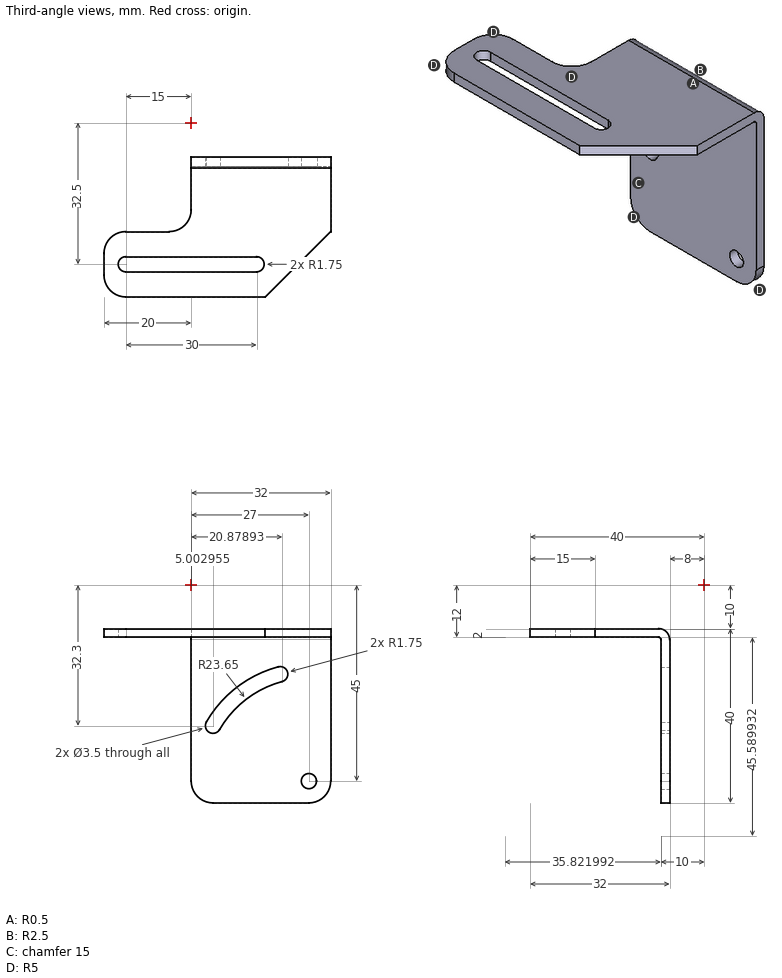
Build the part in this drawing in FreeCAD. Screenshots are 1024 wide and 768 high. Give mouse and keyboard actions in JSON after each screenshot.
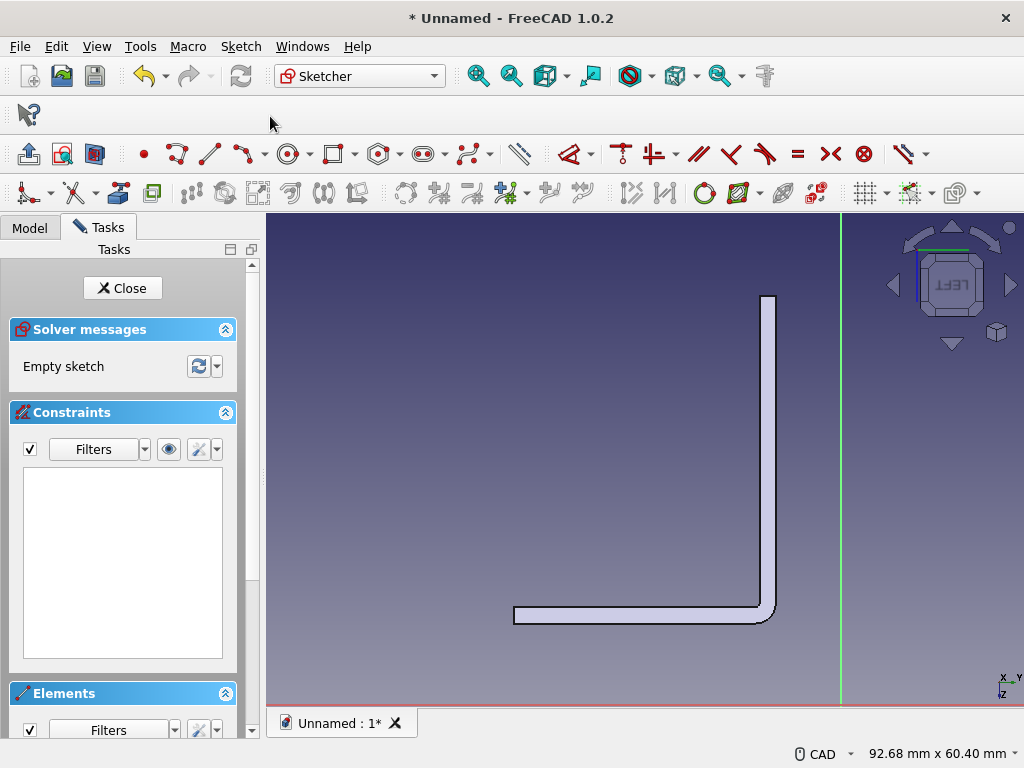
{"action": "scroll", "coordinate": [575, 679], "scroll_direction": "up", "scroll_amount": 6}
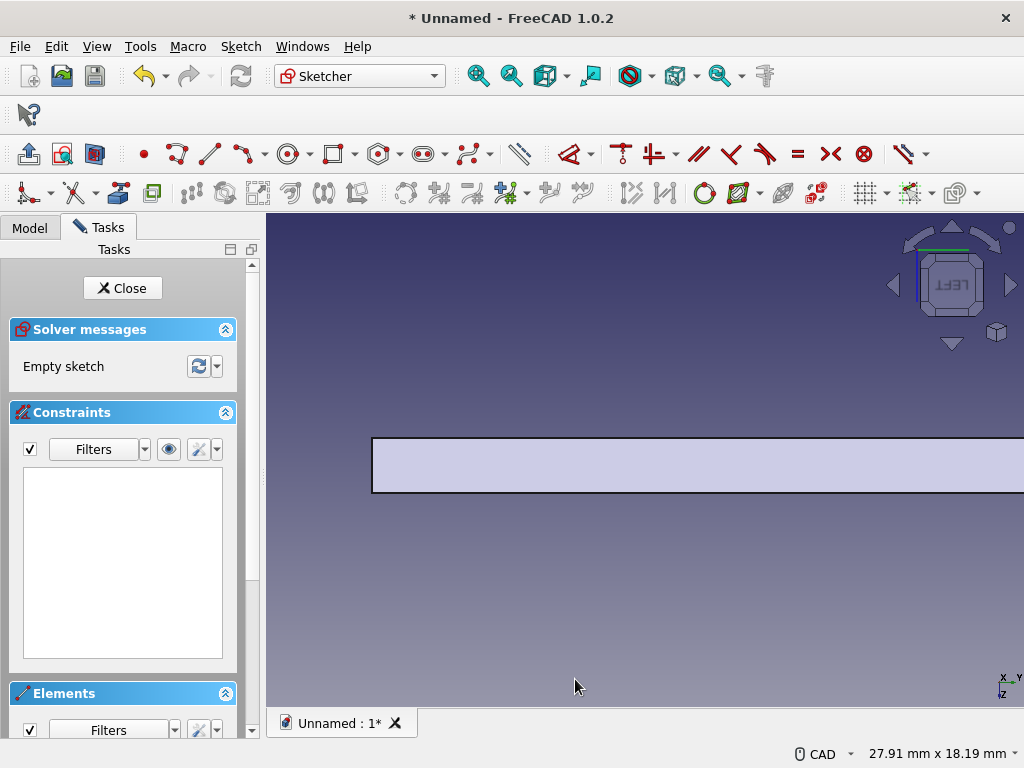
{"action": "left_click", "coordinate": [332, 154]}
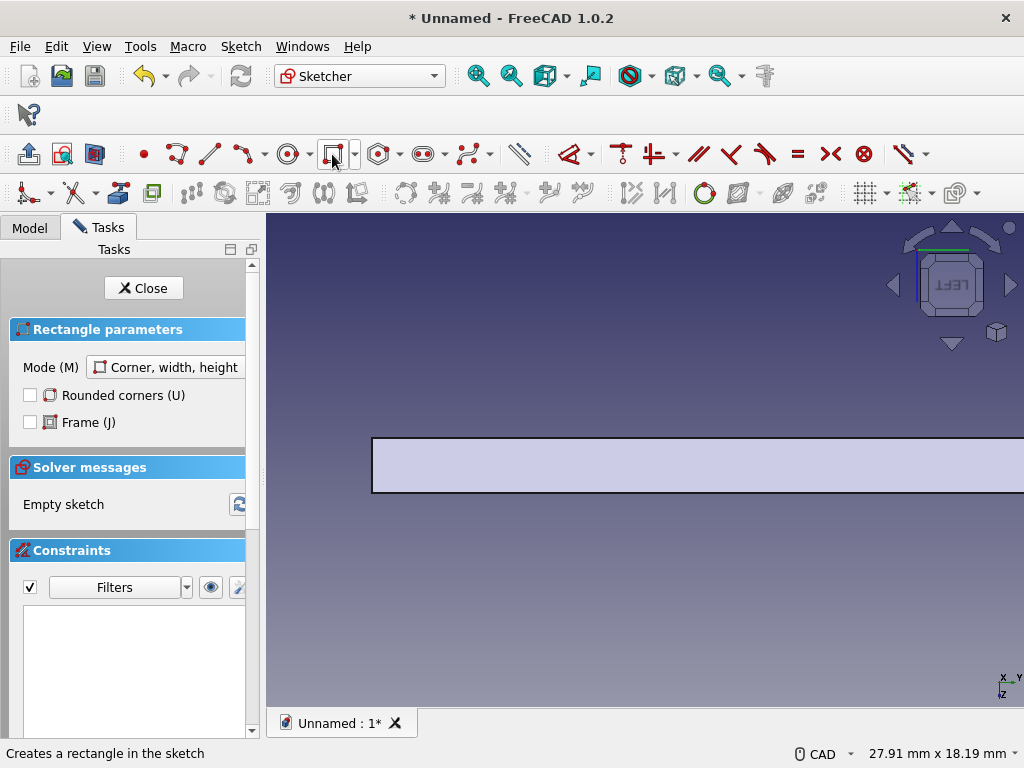
{"action": "left_click", "coordinate": [372, 438]}
{"action": "mouse_move", "coordinate": [779, 493]}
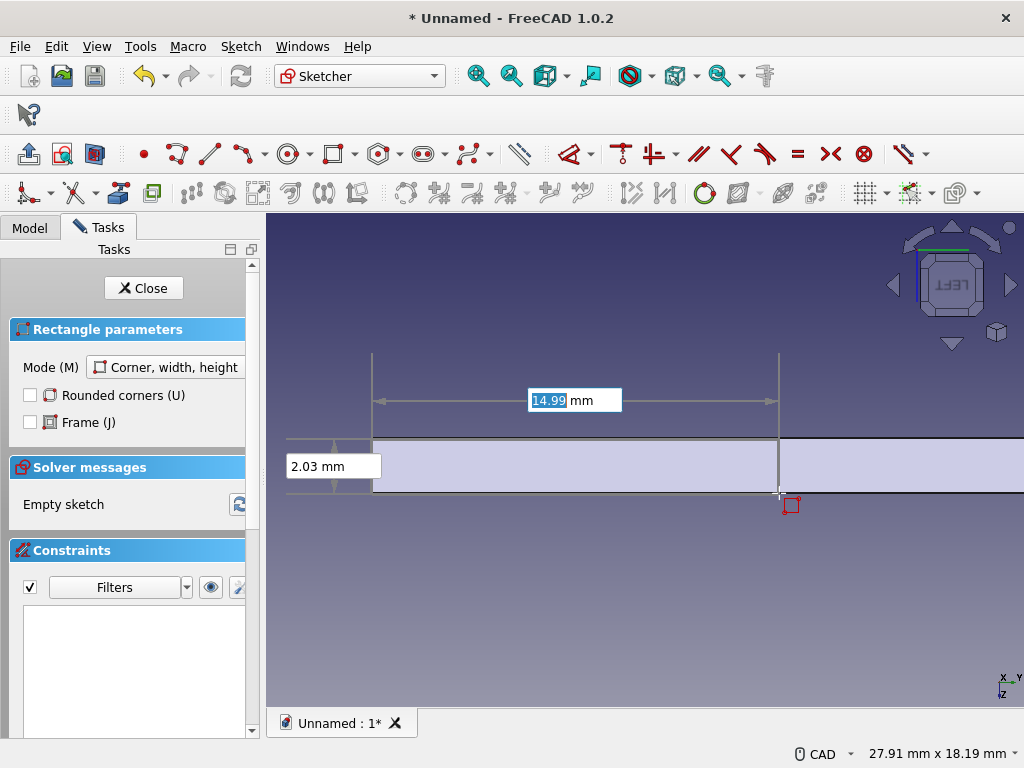
{"action": "type", "text": "15"}
{"action": "key", "text": "Tab"}
{"action": "type", "text": "2"}
{"action": "key", "text": "Return"}
{"action": "key", "text": "Escape"}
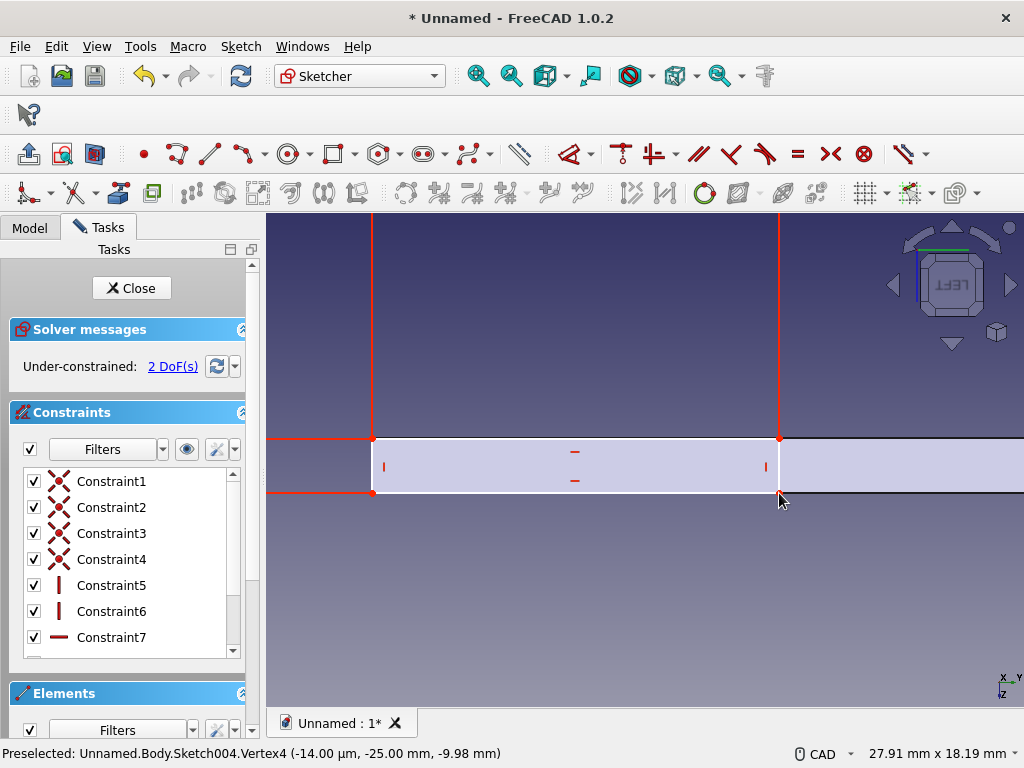
{"action": "key", "text": "d"}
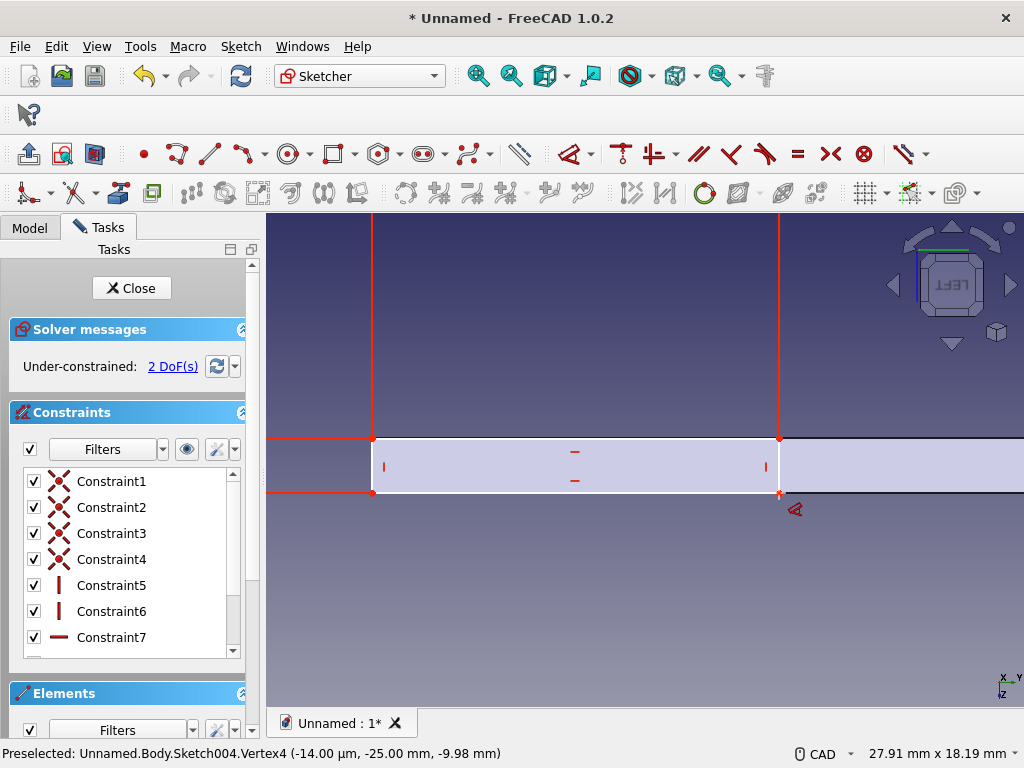
{"action": "left_click", "coordinate": [372, 439]}
{"action": "left_click", "coordinate": [616, 405]}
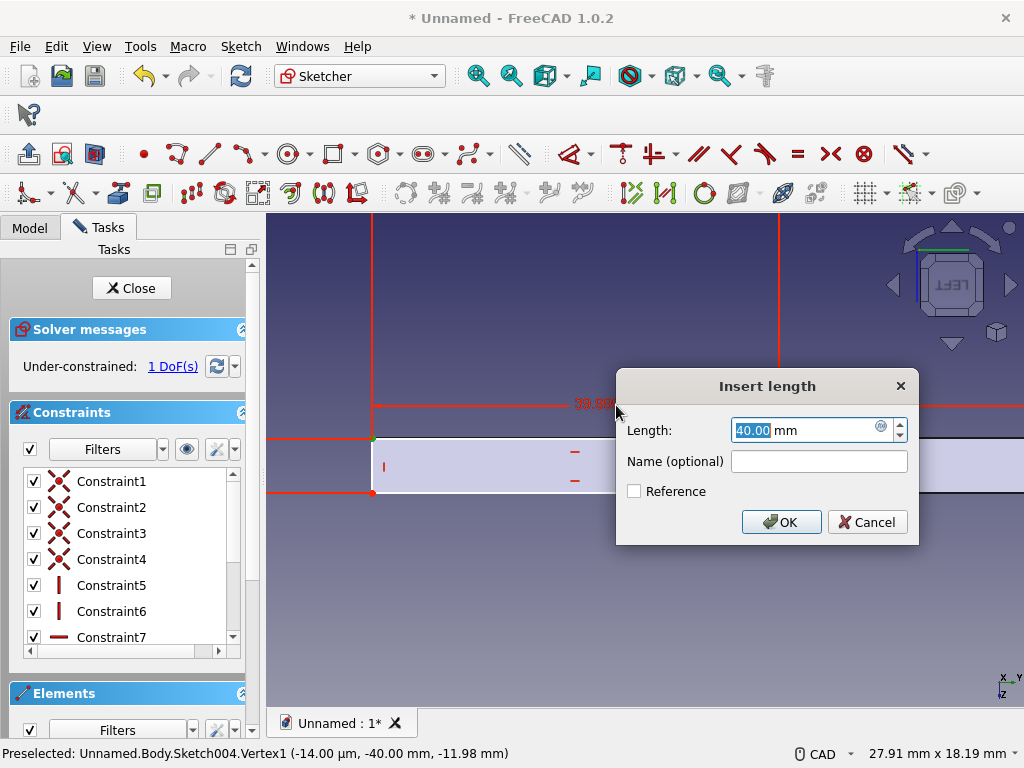
{"action": "type", "text": "40"}
{"action": "key", "text": "Return"}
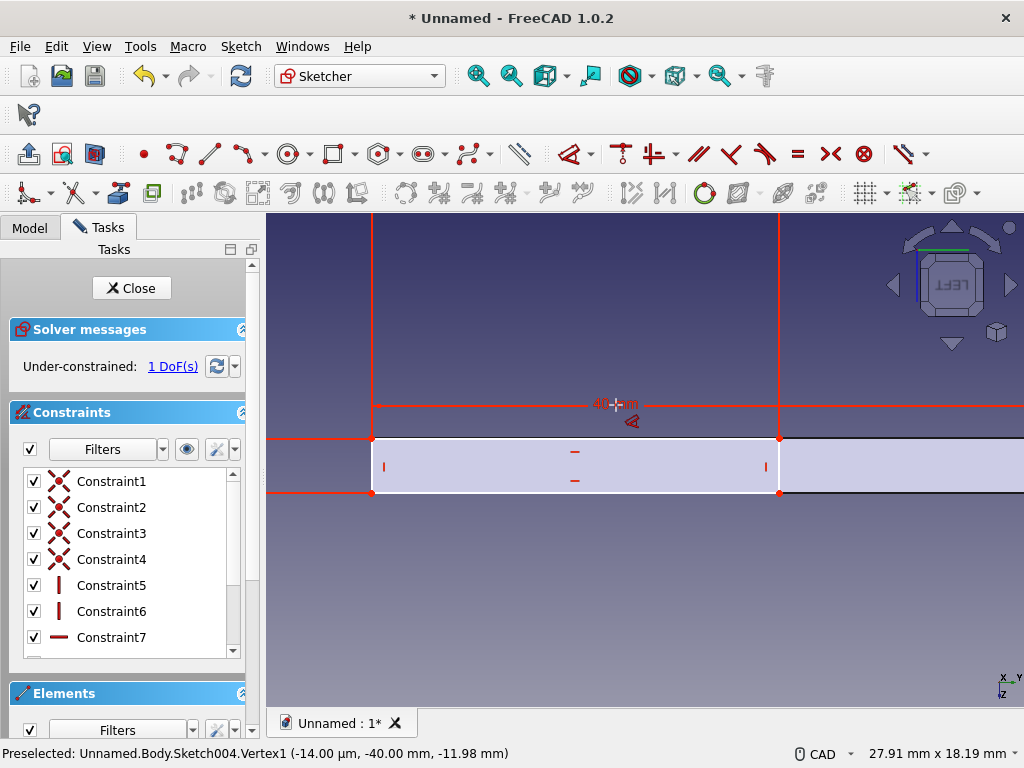
{"action": "left_click", "coordinate": [372, 439]}
{"action": "left_click", "coordinate": [338, 559]}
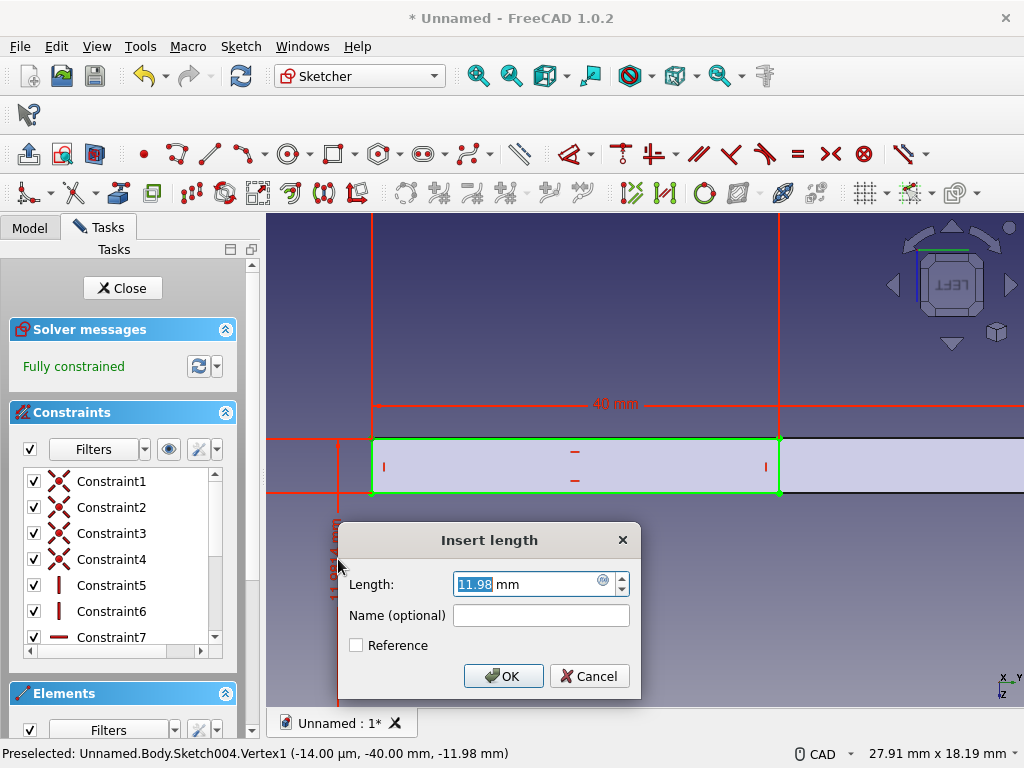
{"action": "type", "text": "12"}
{"action": "key", "text": "Return"}
{"action": "key", "text": "Escape"}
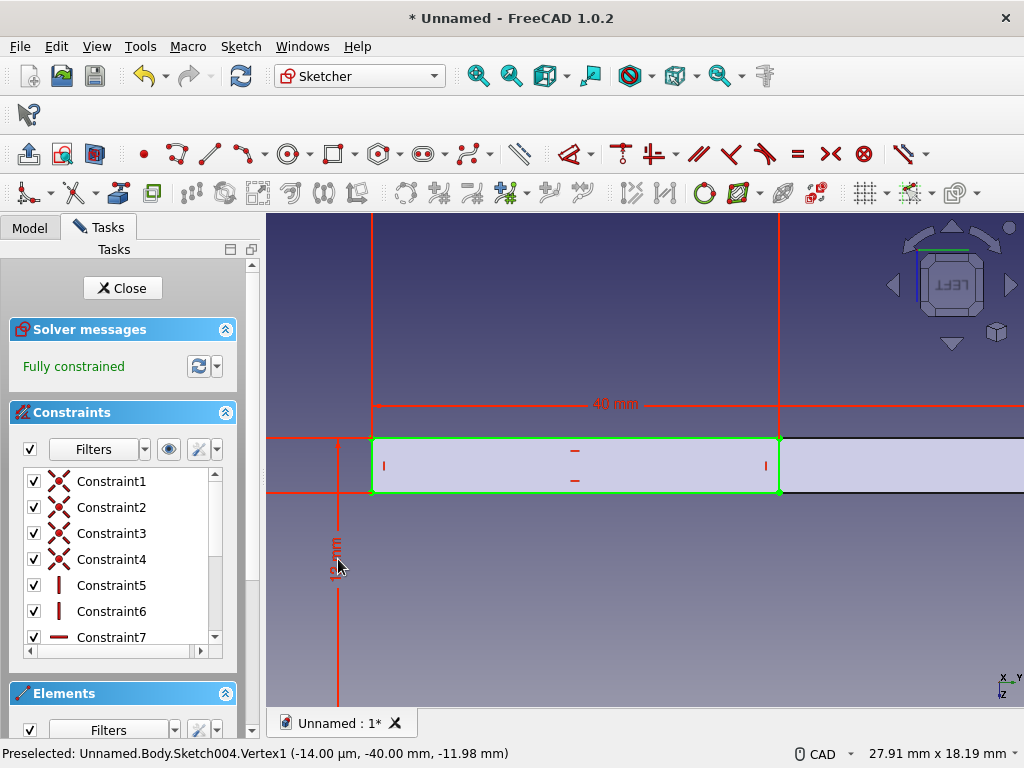
{"action": "left_click", "coordinate": [123, 288]}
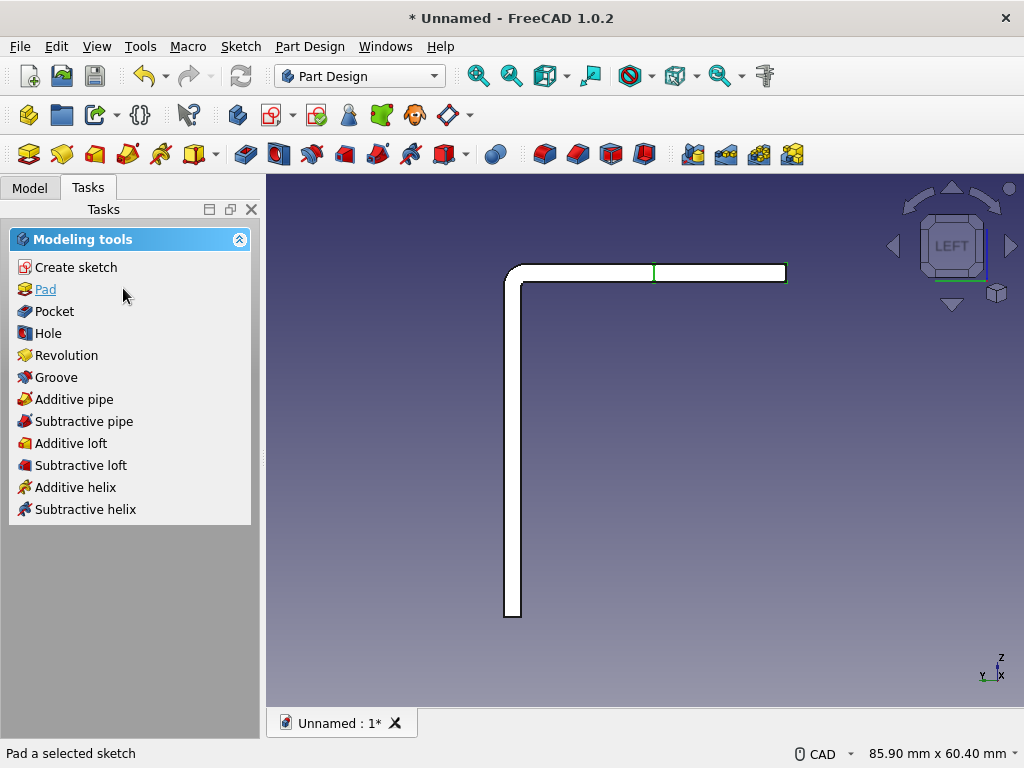
{"action": "left_click", "coordinate": [29, 154]}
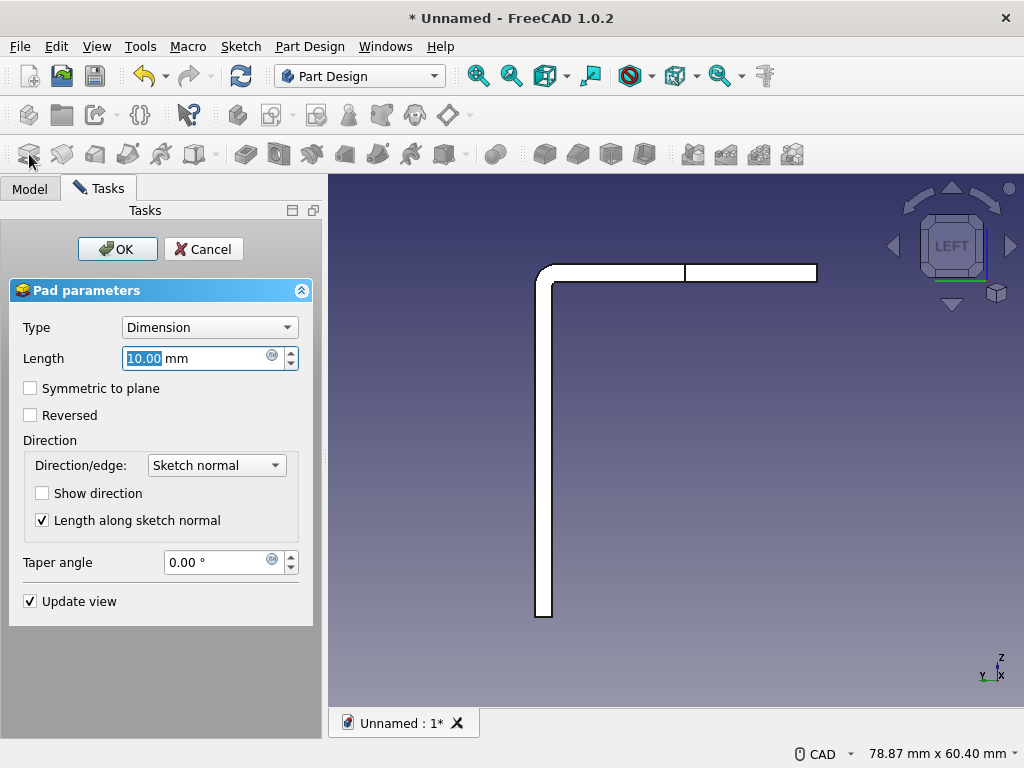
{"action": "type", "text": "20"}
{"action": "key", "text": "Tab"}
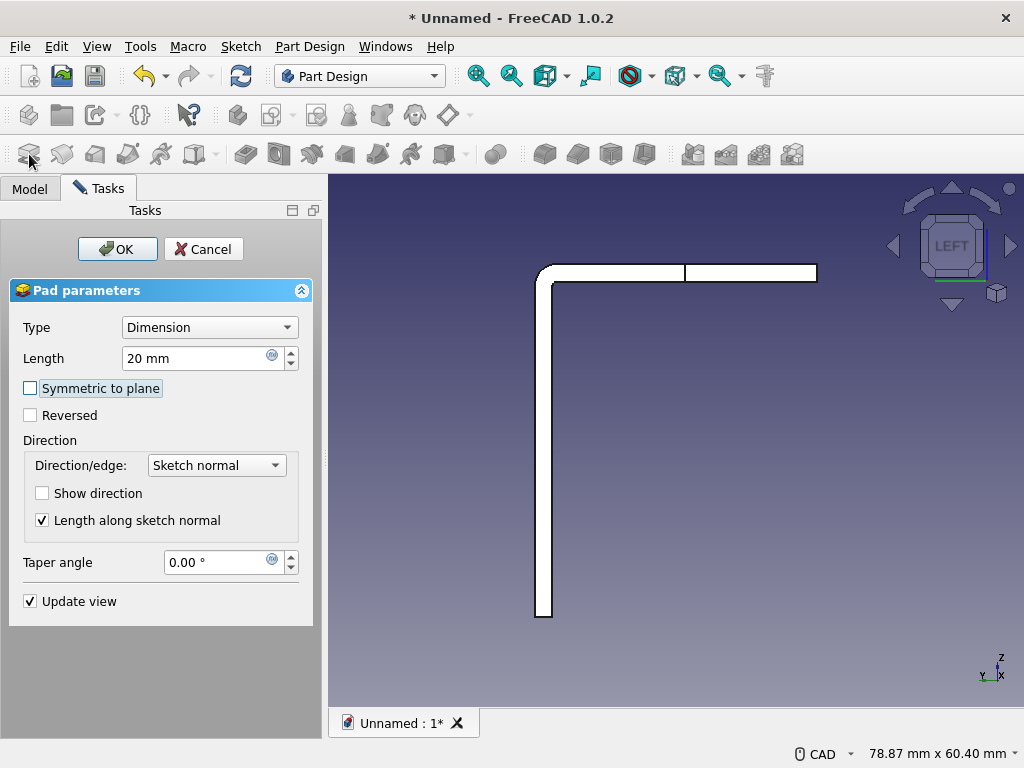
{"action": "left_click", "coordinate": [118, 249]}